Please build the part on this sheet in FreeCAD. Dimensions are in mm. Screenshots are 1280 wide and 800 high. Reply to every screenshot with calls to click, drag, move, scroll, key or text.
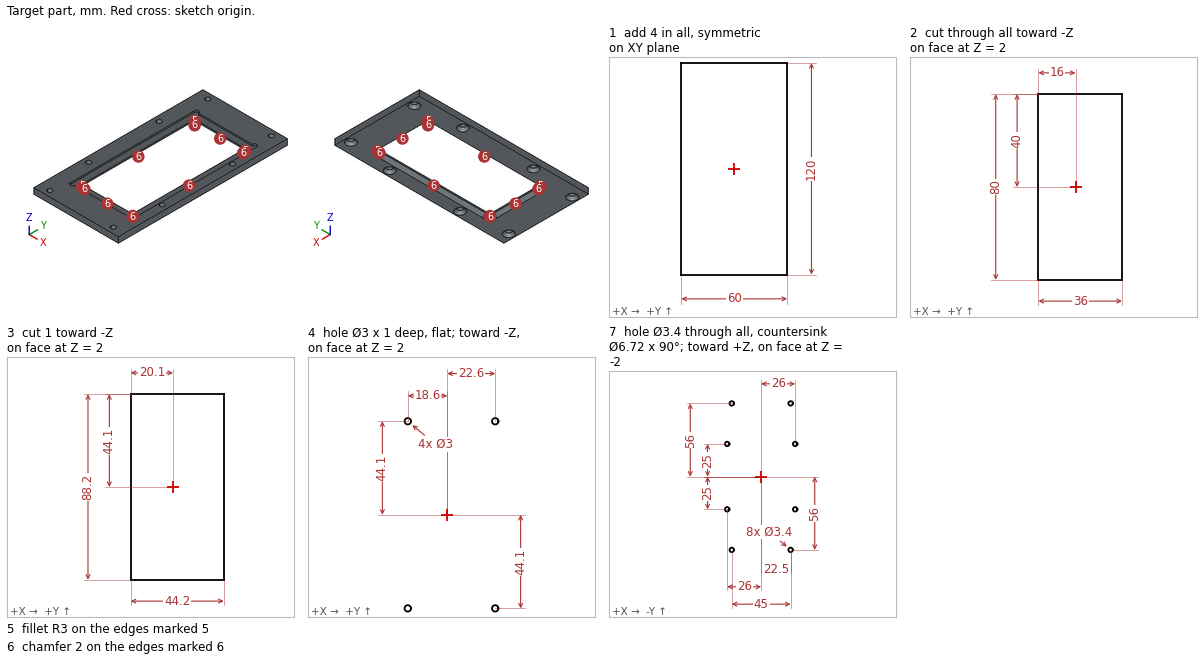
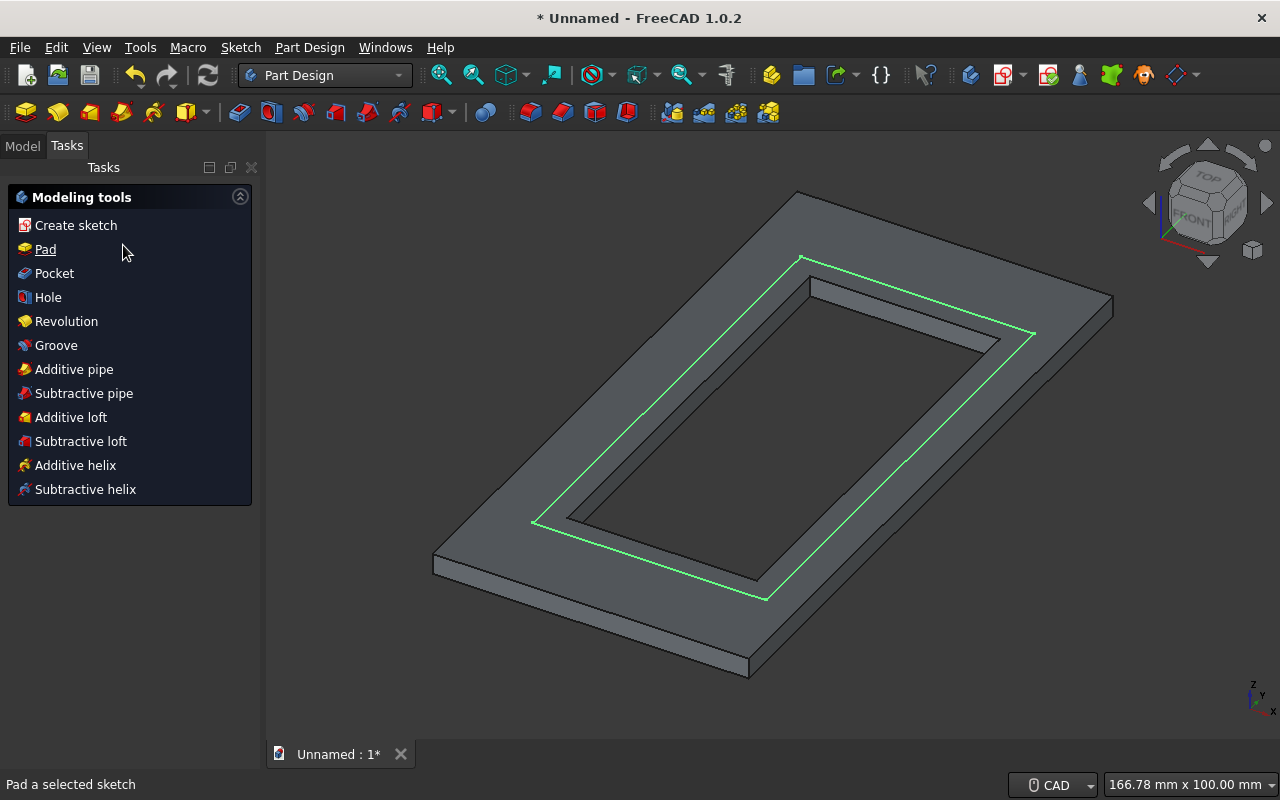
click(240, 112)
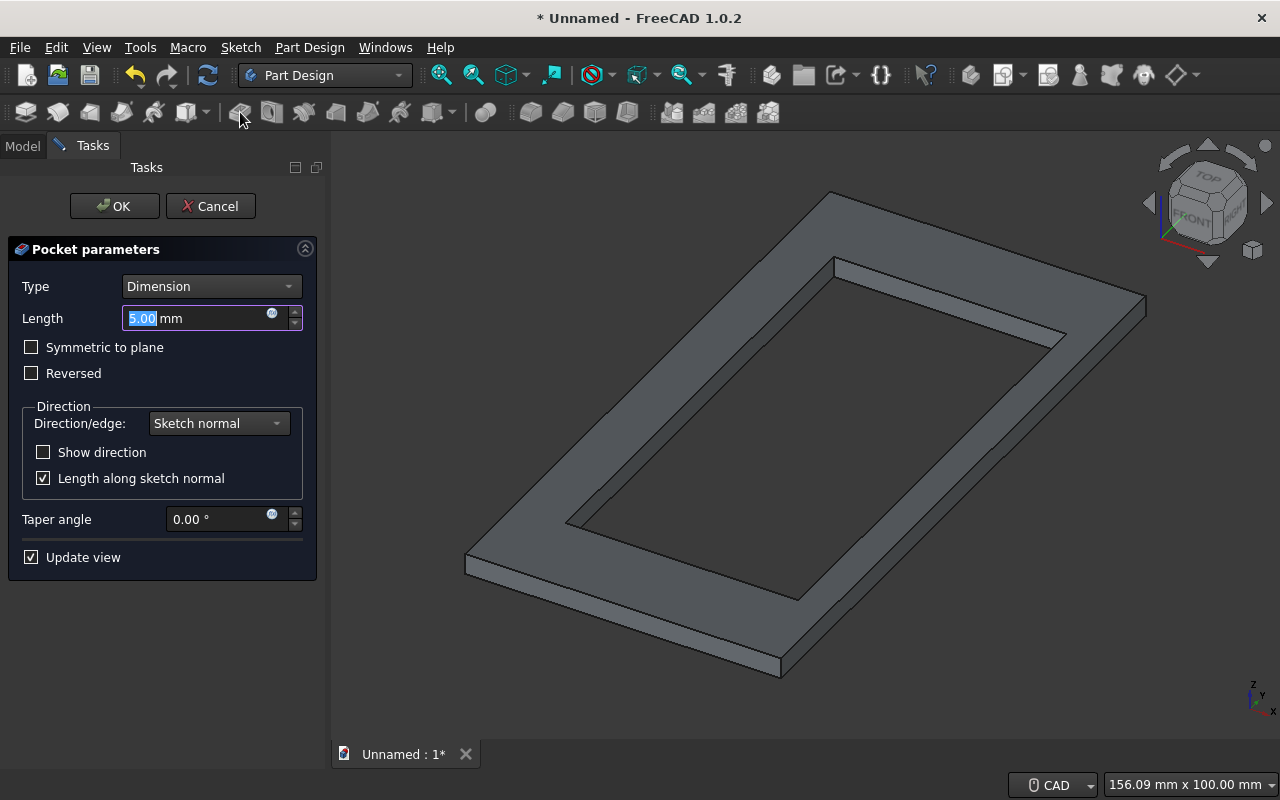
text(1)
key(Tab)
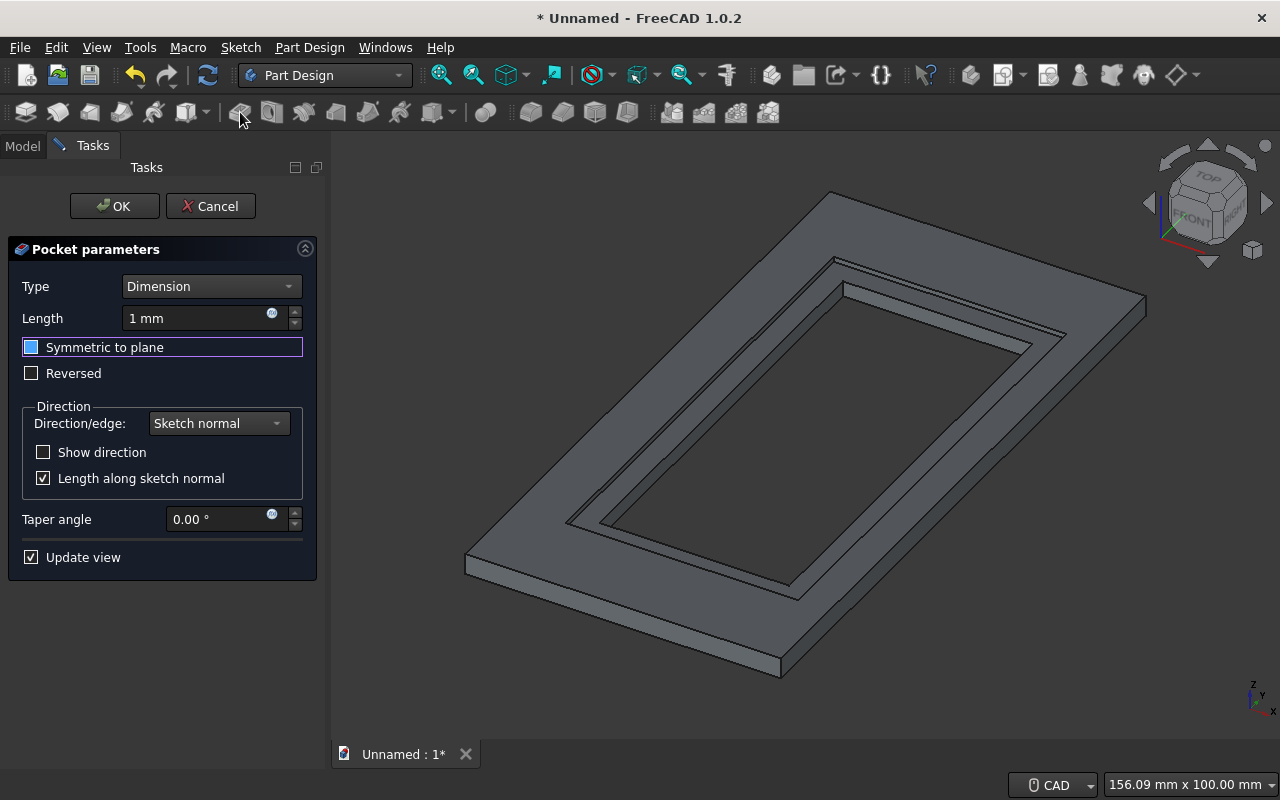
click(115, 206)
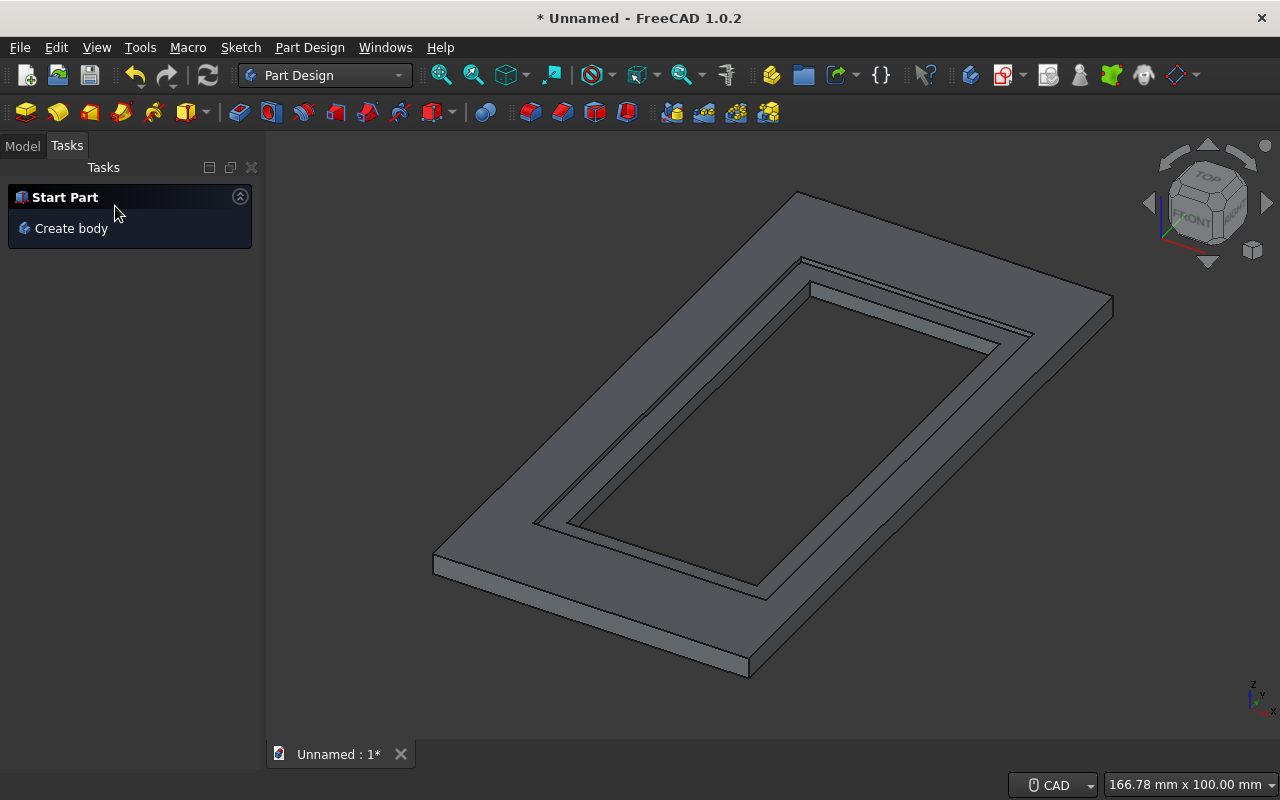
click(707, 609)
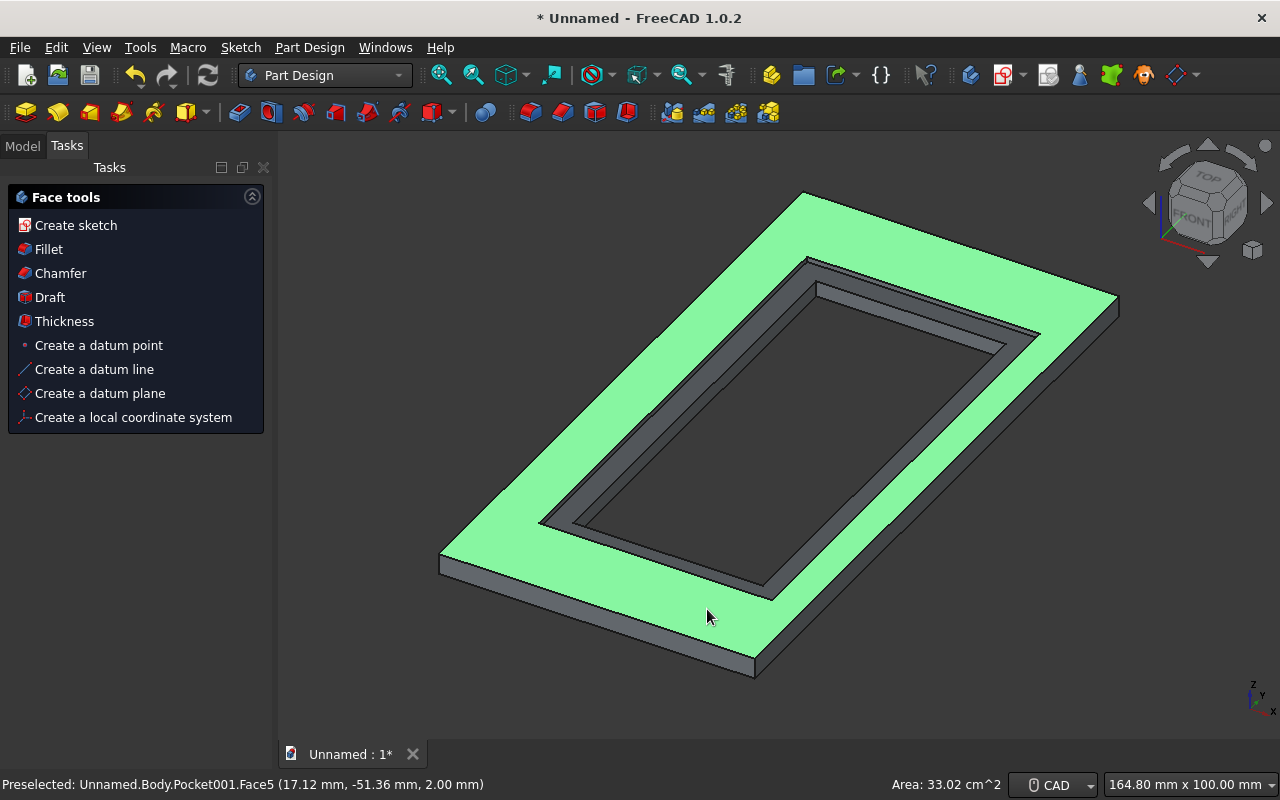
click(1004, 76)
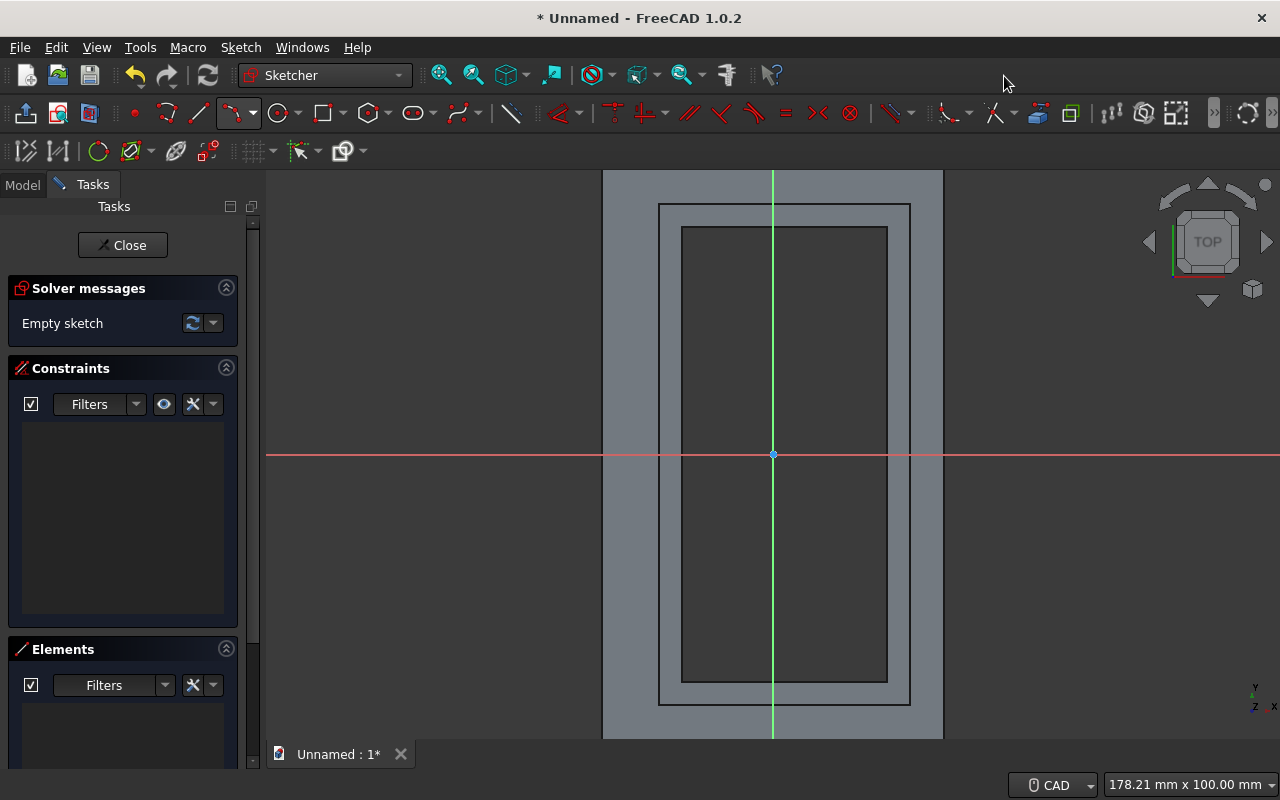
scroll(542, 455, down, 2)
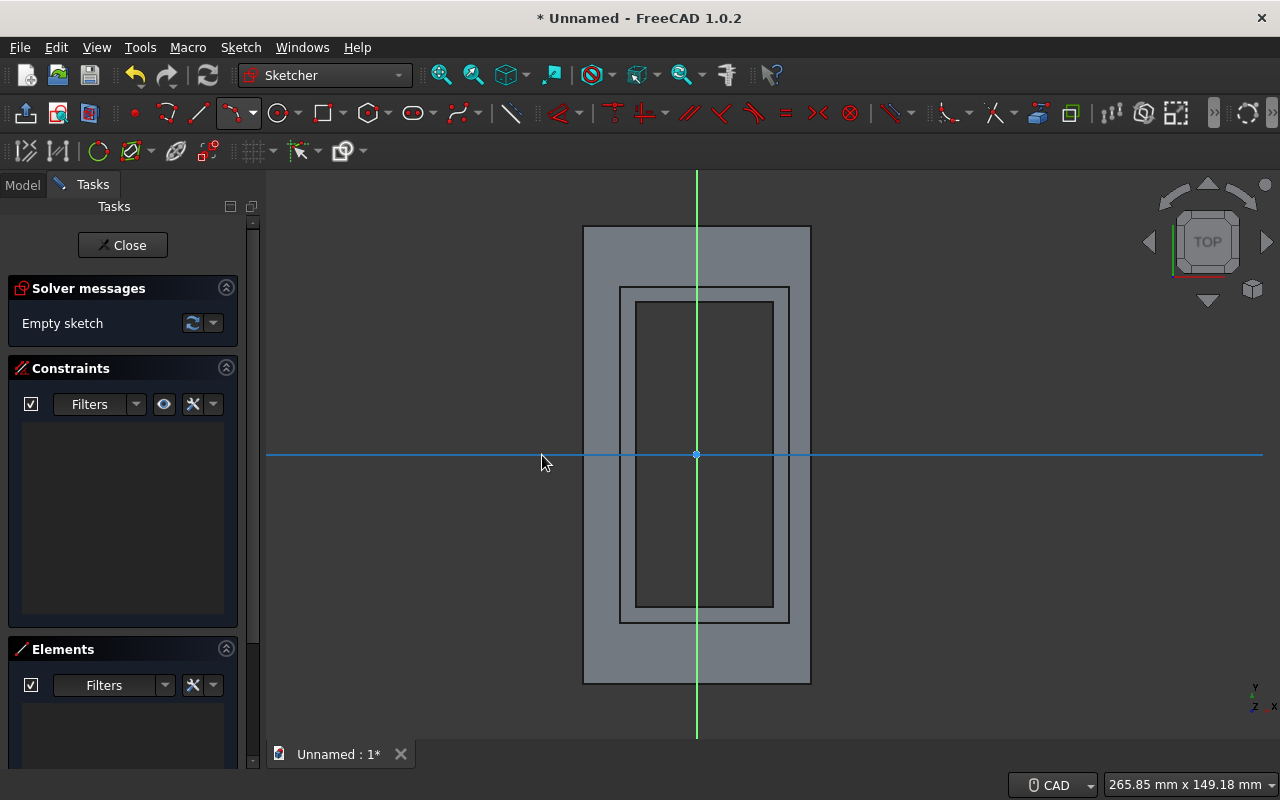
click(278, 114)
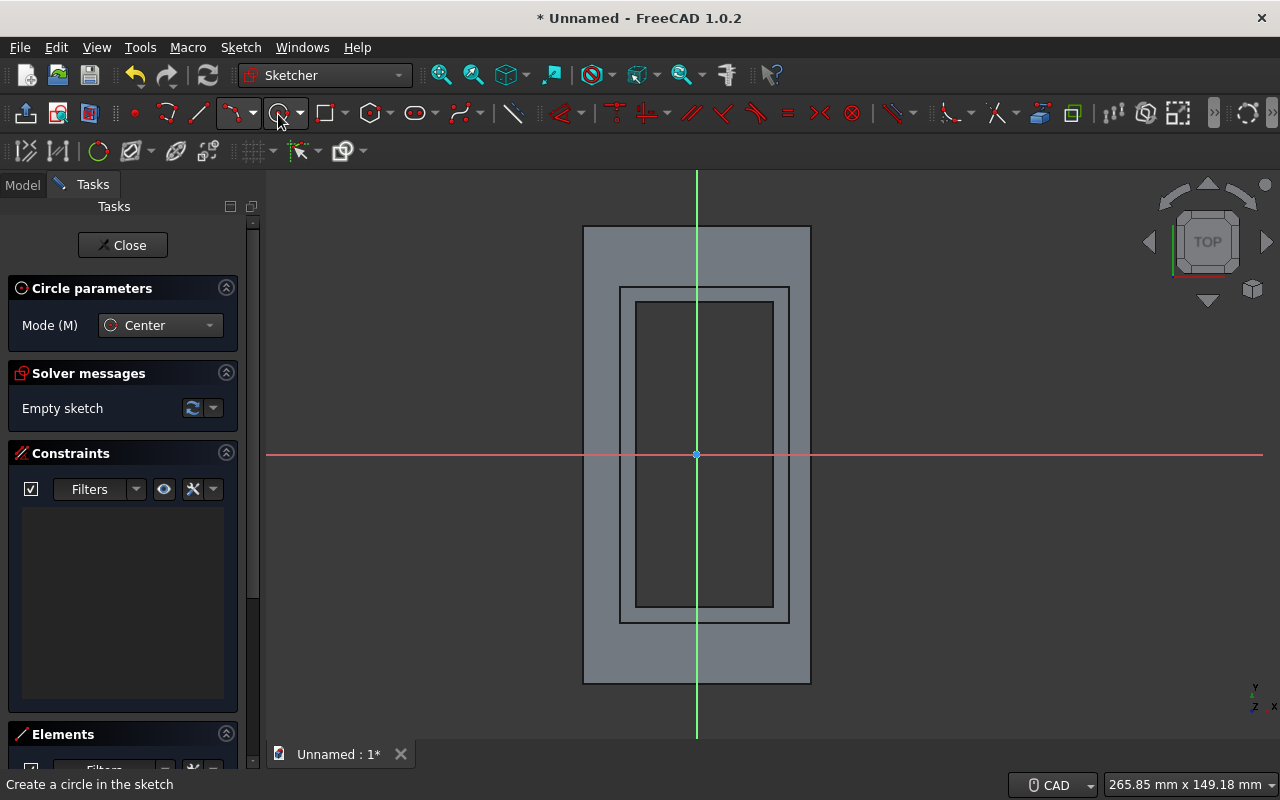
scroll(626, 287, up, 7)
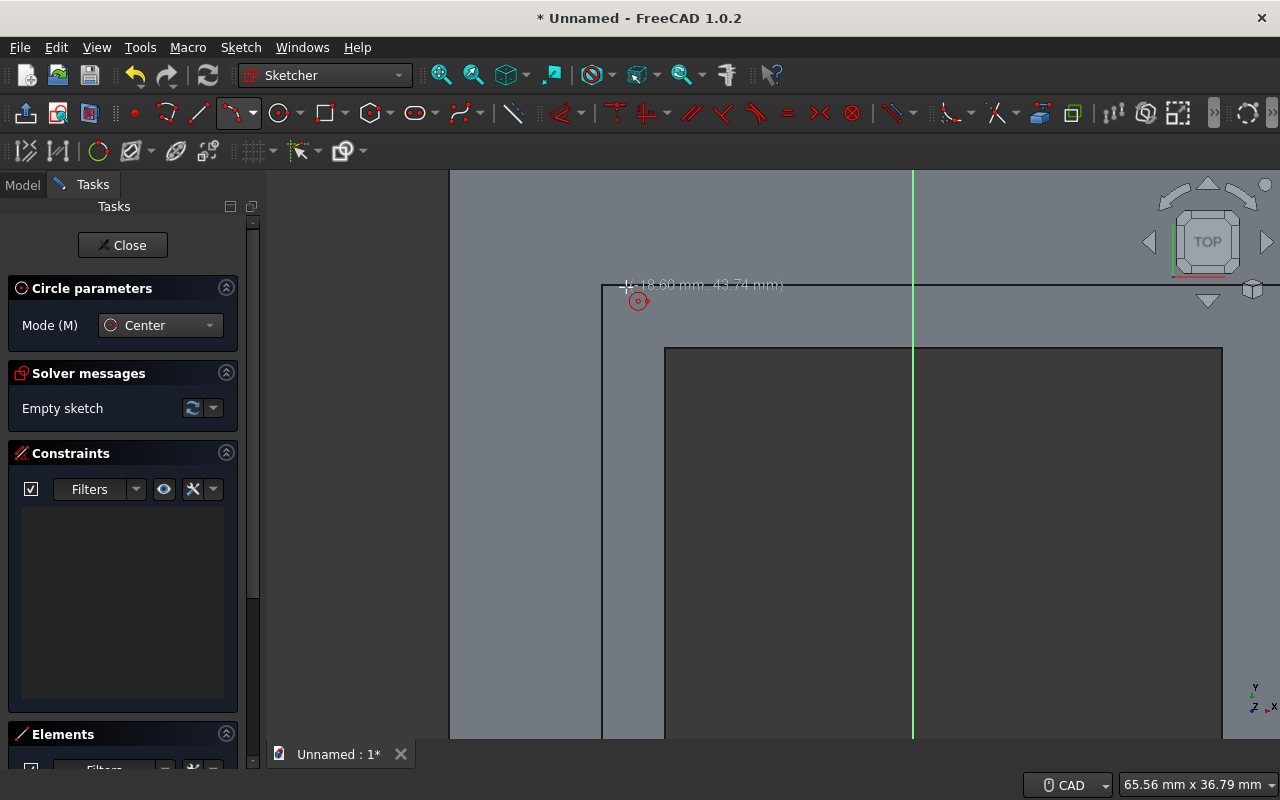
scroll(626, 287, down, 7)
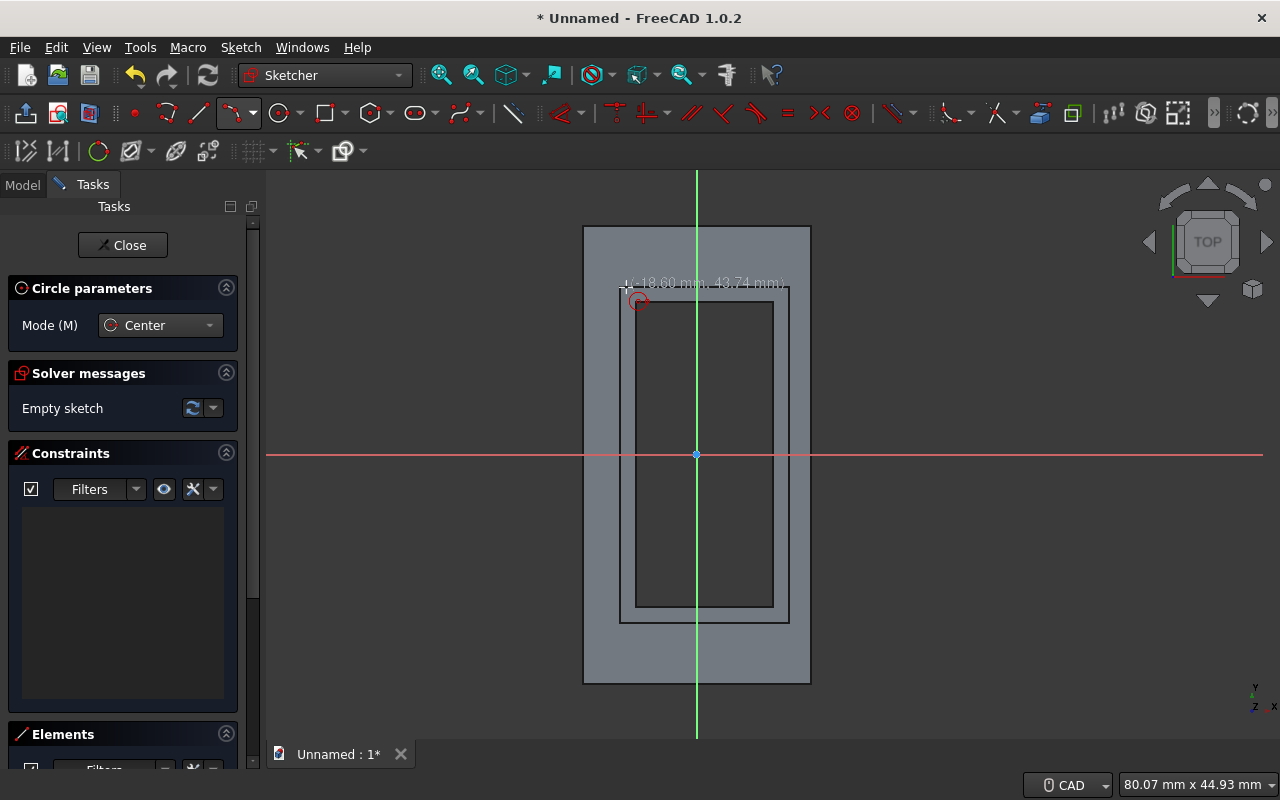
click(626, 287)